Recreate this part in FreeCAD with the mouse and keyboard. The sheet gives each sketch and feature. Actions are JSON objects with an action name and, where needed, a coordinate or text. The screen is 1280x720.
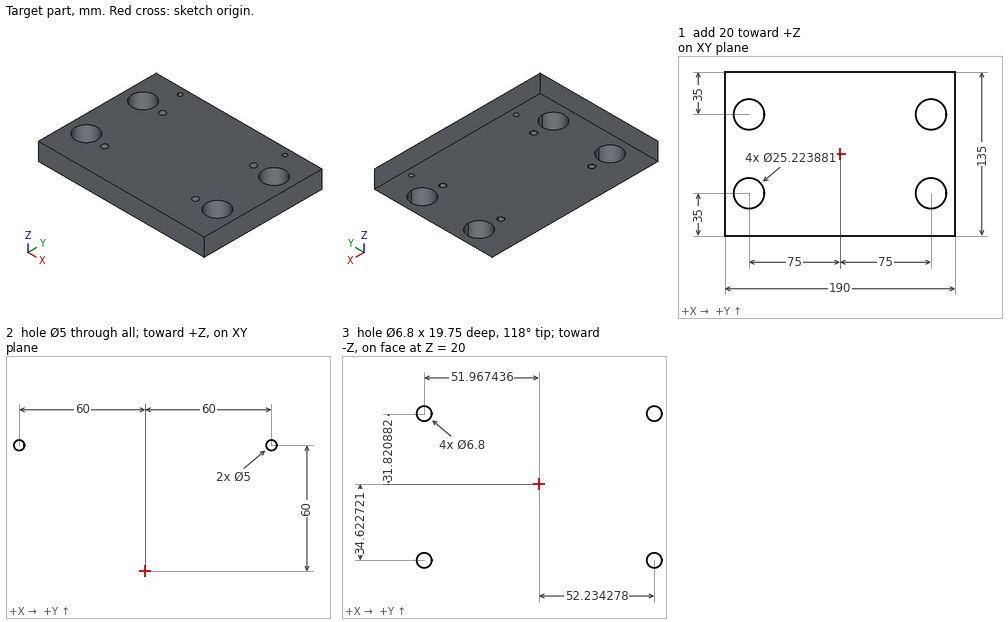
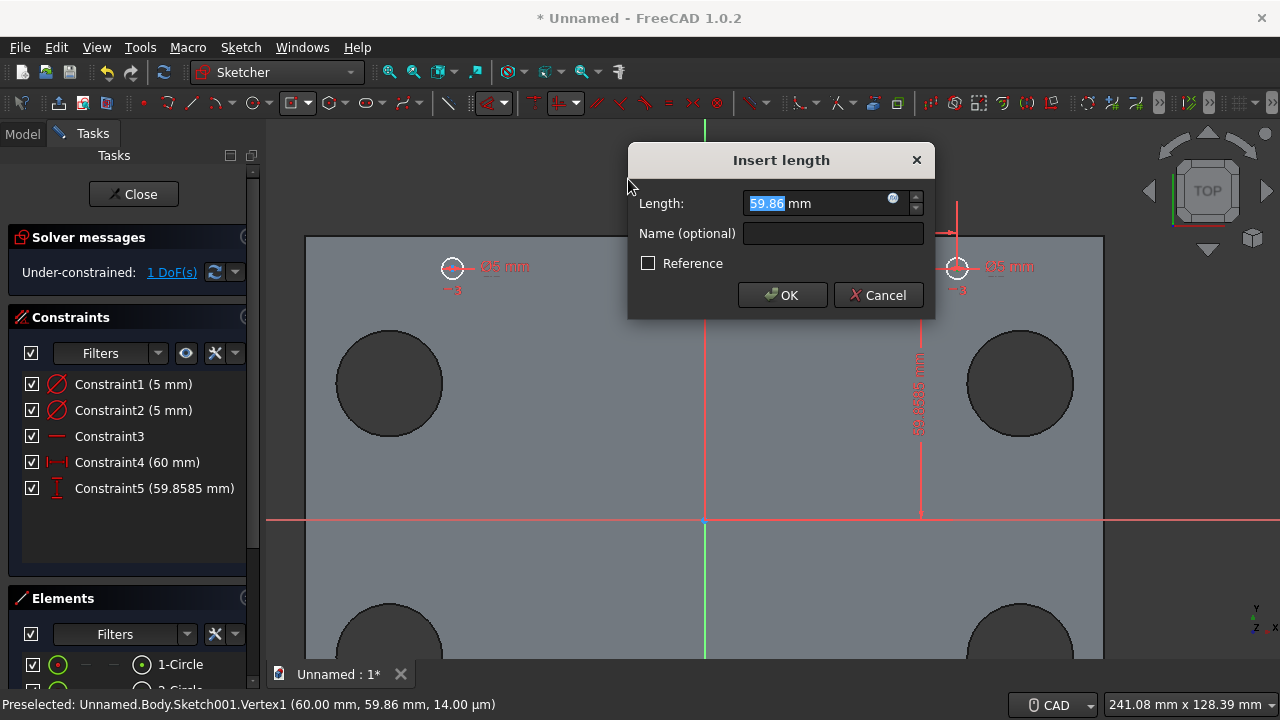
{"action": "type", "text": "60"}
{"action": "key", "text": "Return"}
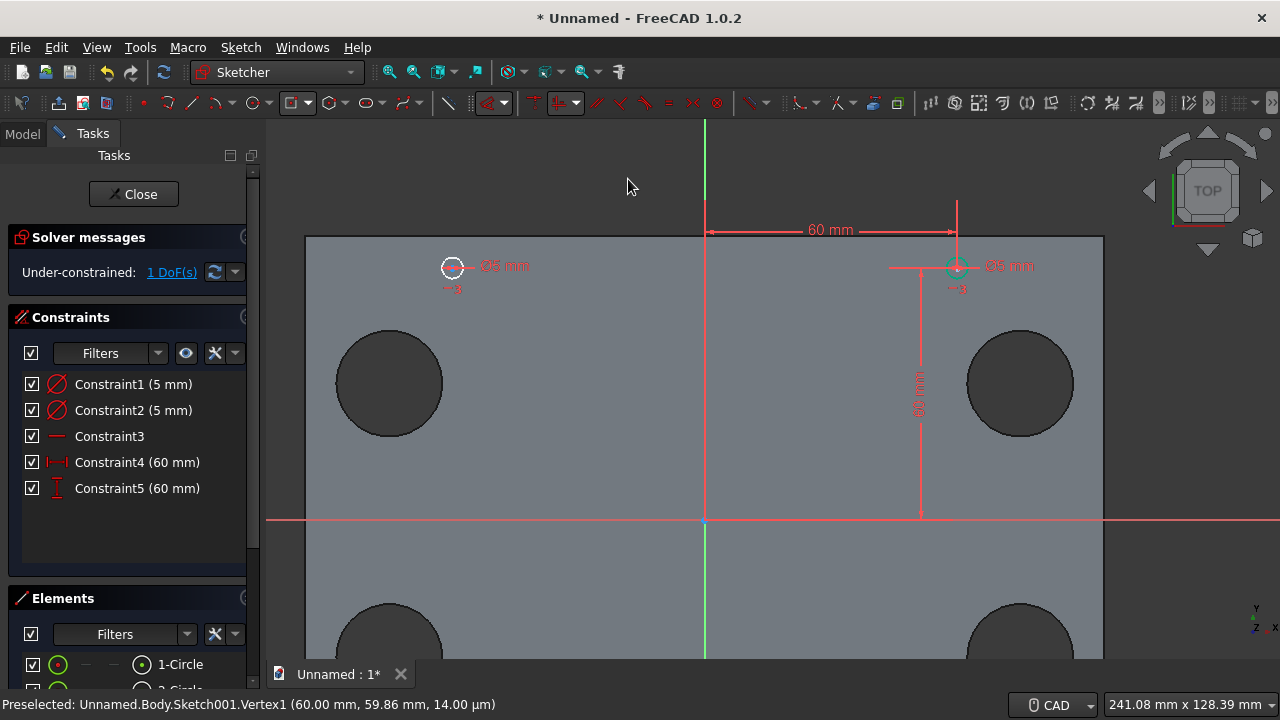
{"action": "left_click", "coordinate": [453, 268]}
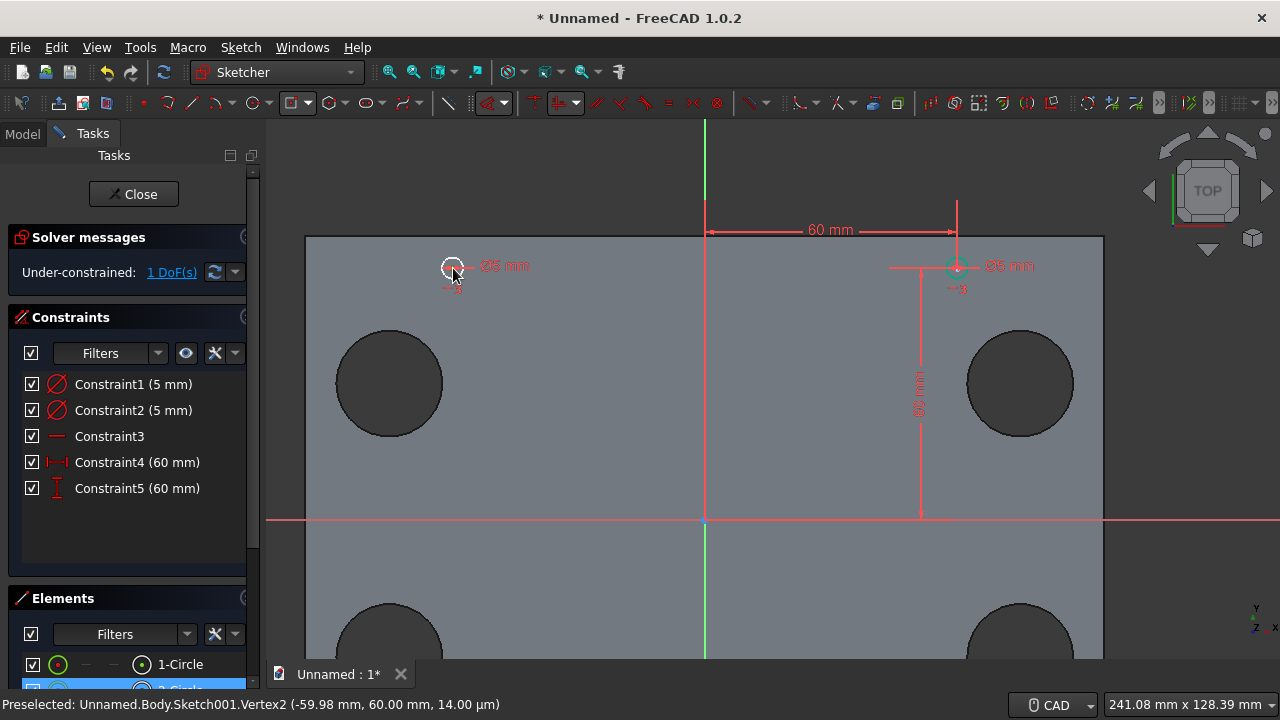
{"action": "left_click", "coordinate": [506, 104]}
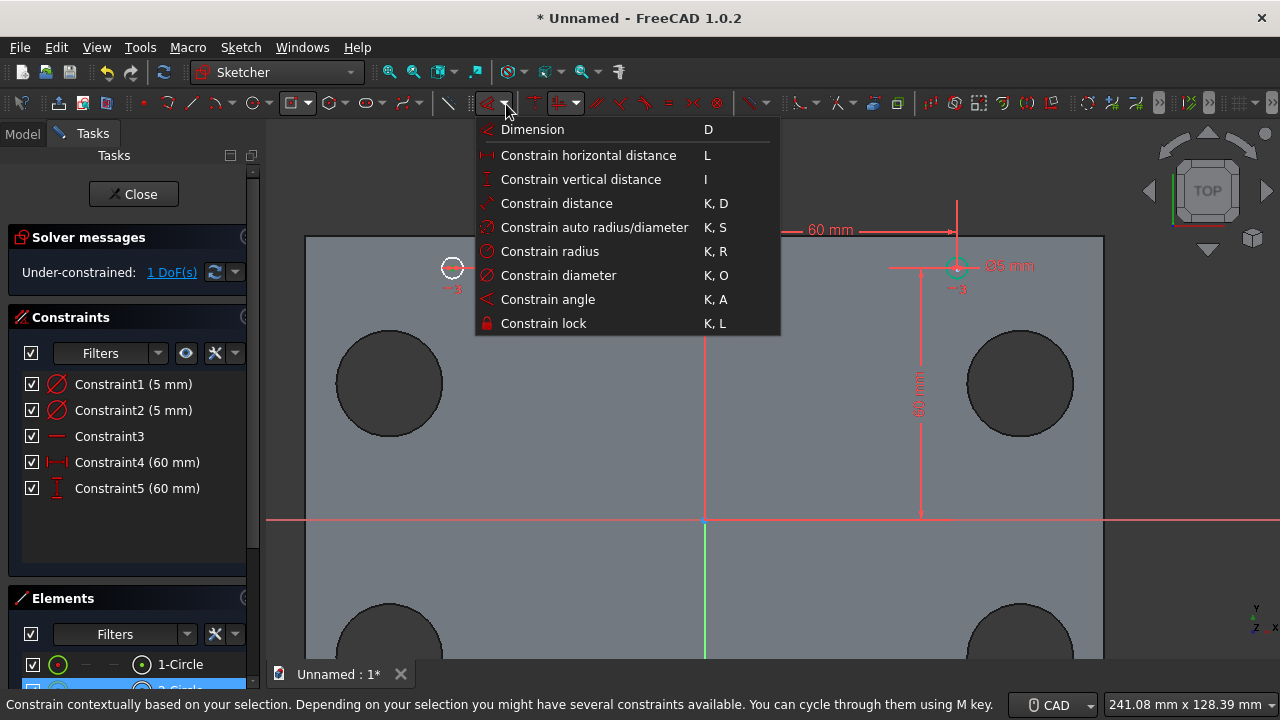
{"action": "left_click", "coordinate": [628, 155]}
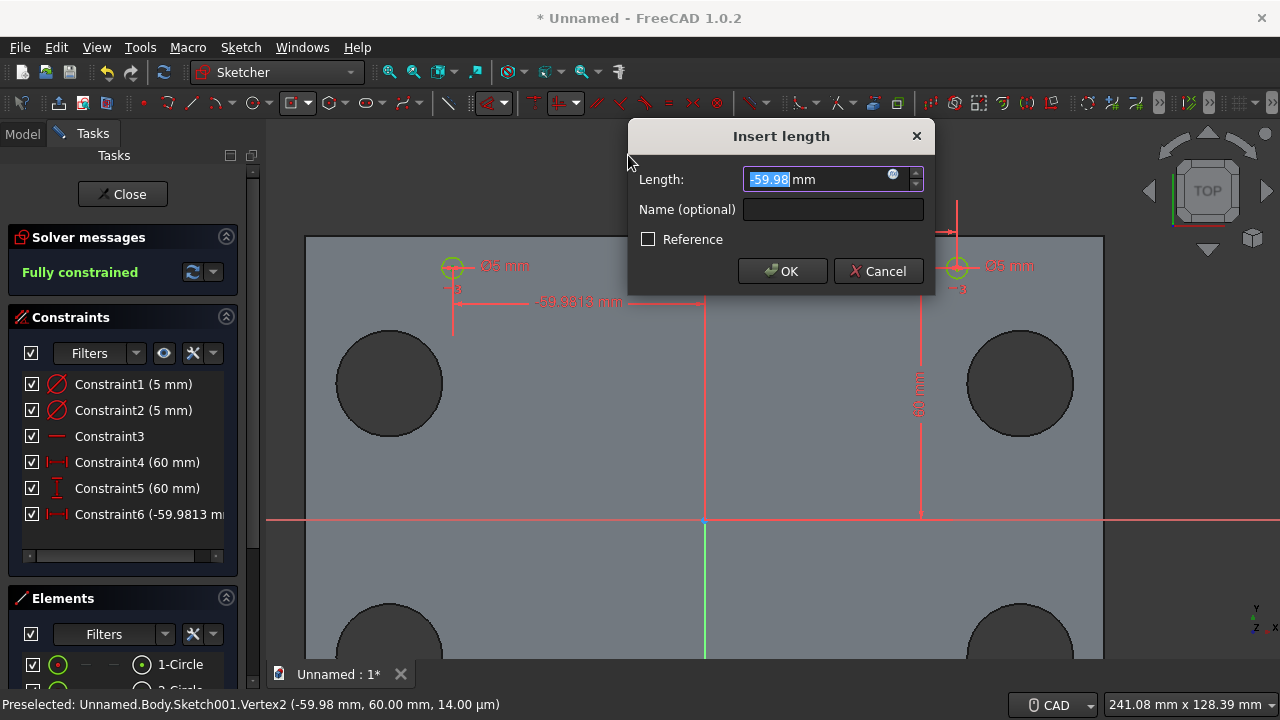
{"action": "type", "text": "-60"}
{"action": "key", "text": "Return"}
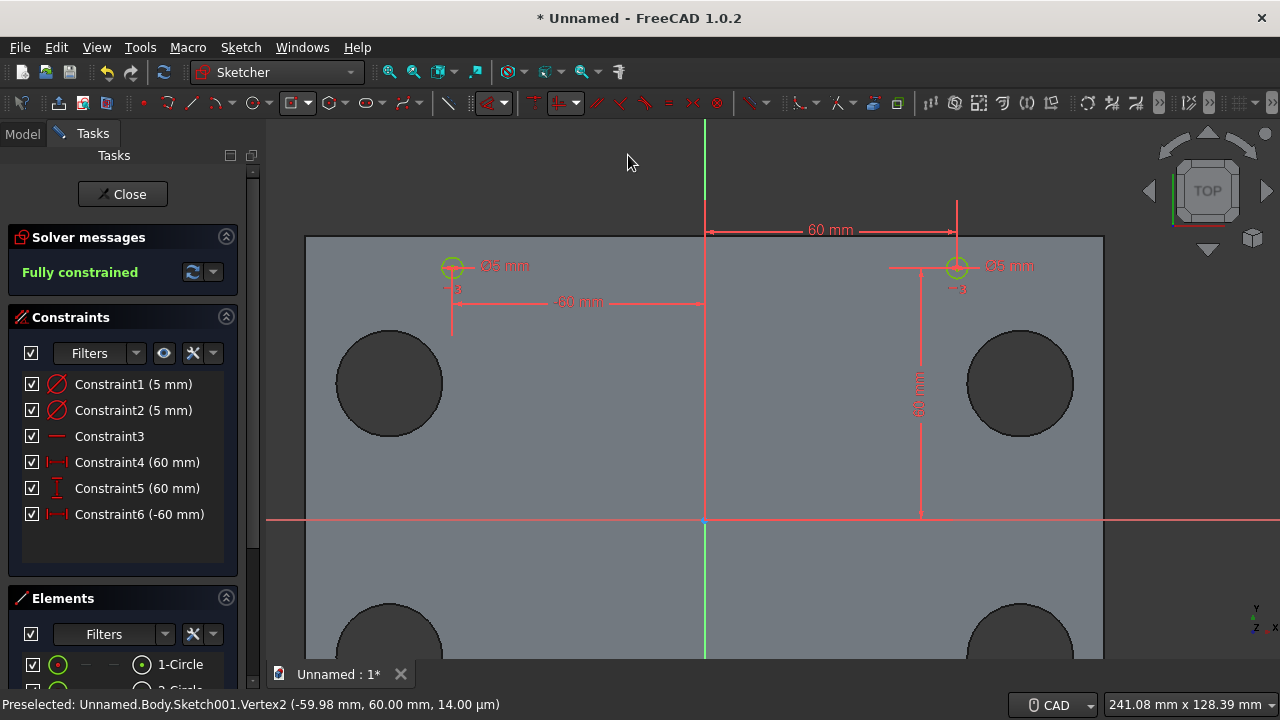
{"action": "left_click", "coordinate": [123, 194]}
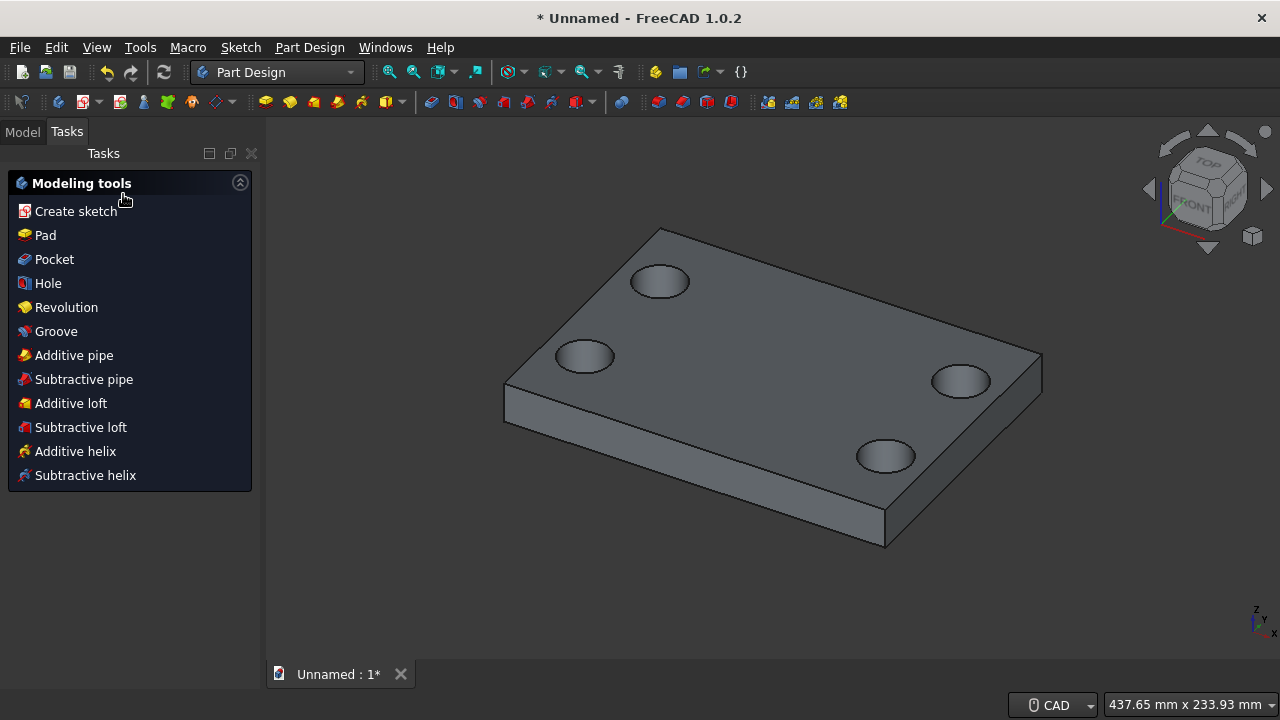
{"action": "left_click", "coordinate": [456, 102]}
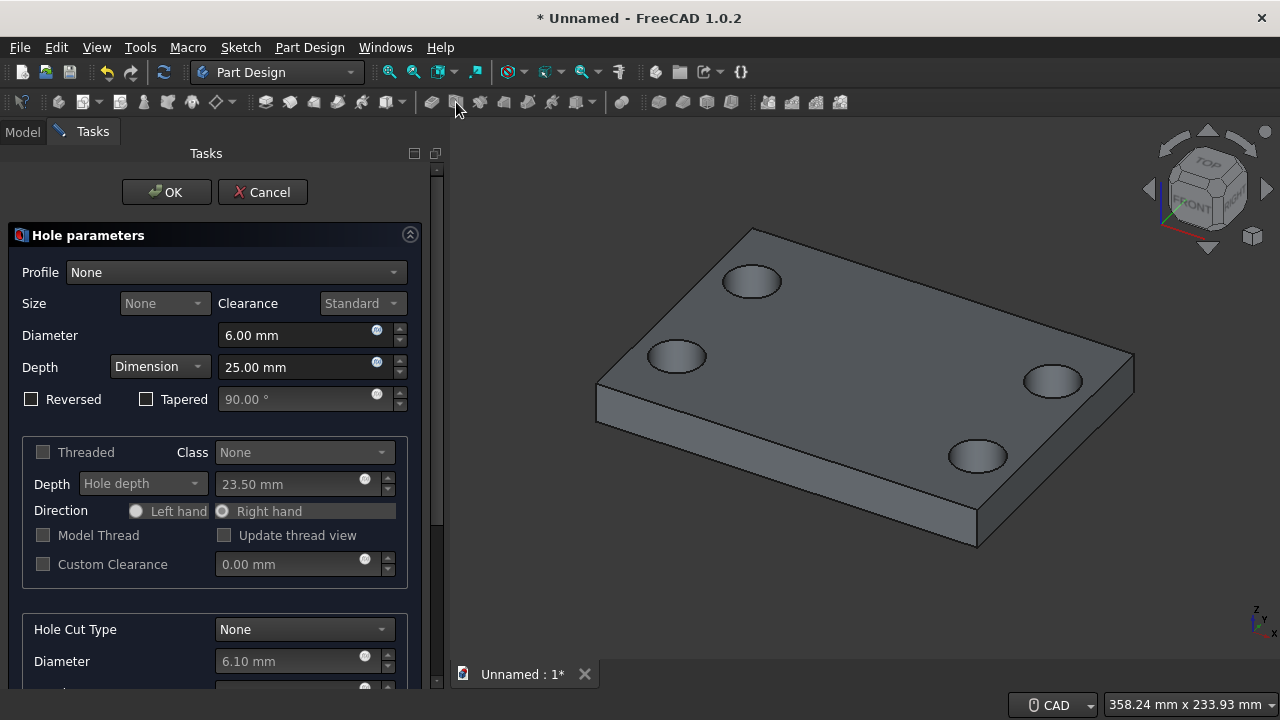
{"action": "triple_click", "coordinate": [305, 335]}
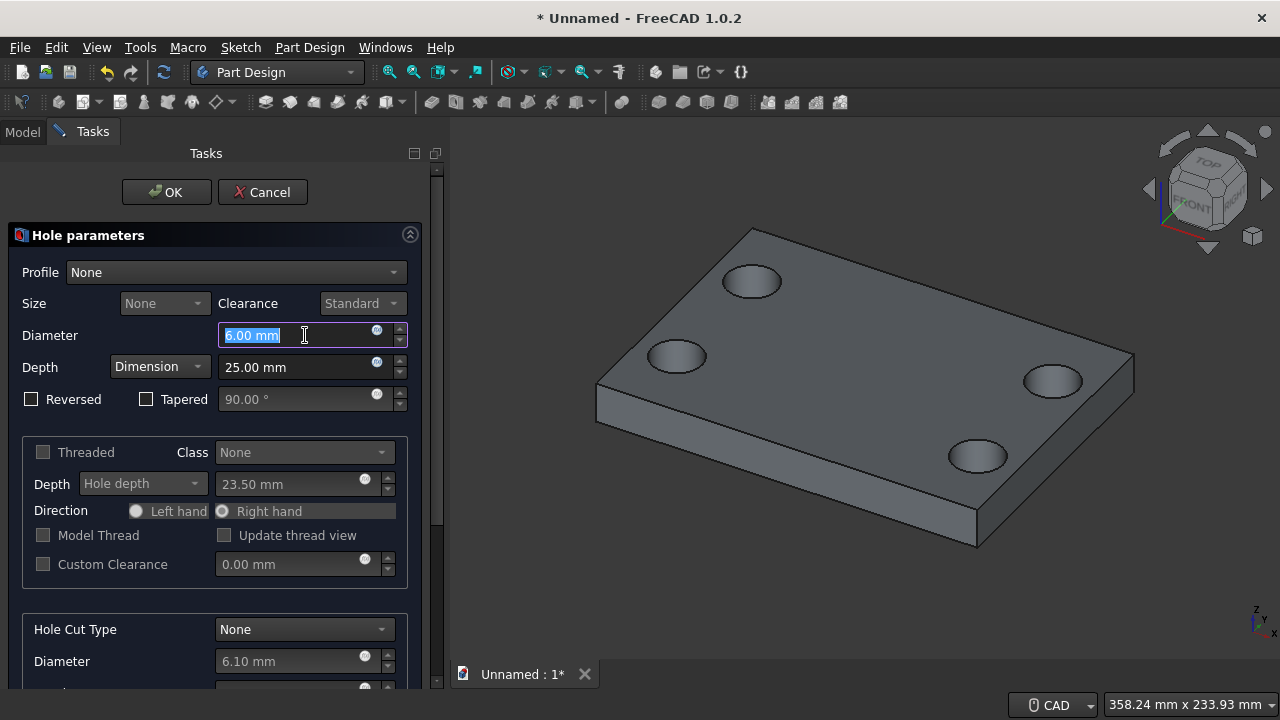
{"action": "type", "text": "5"}
{"action": "key", "text": "Tab"}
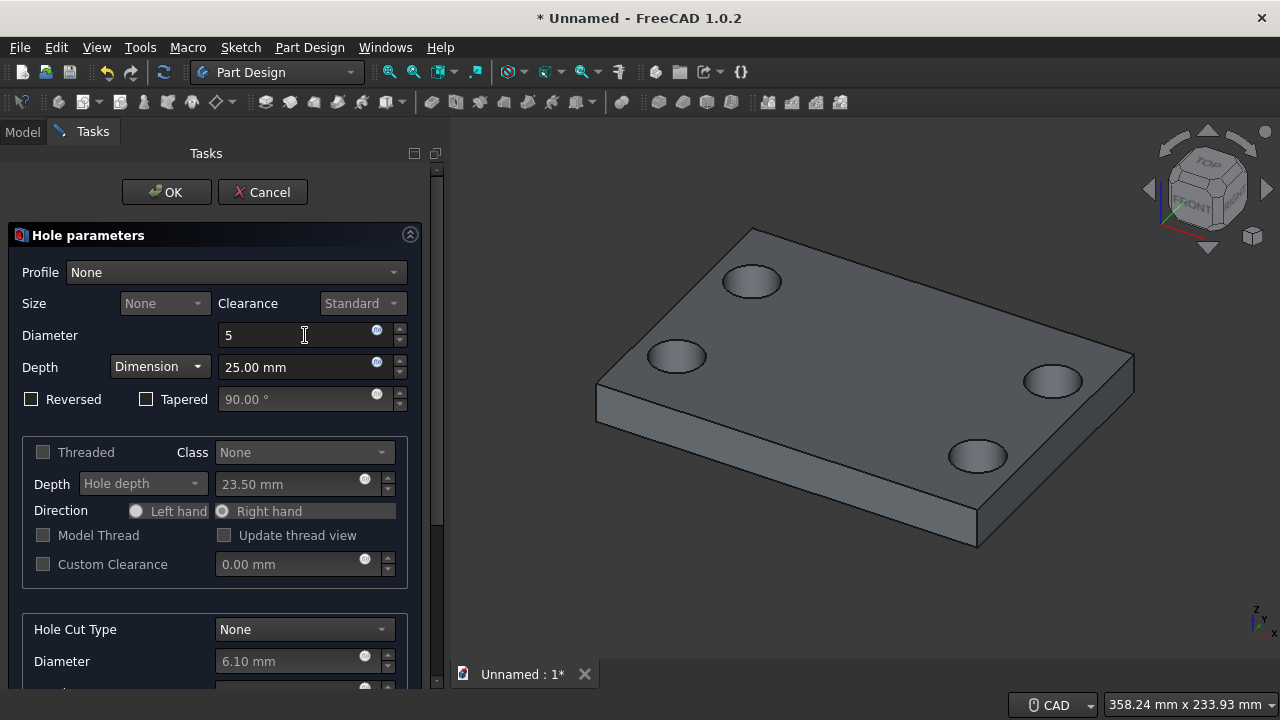
{"action": "left_click", "coordinate": [161, 366]}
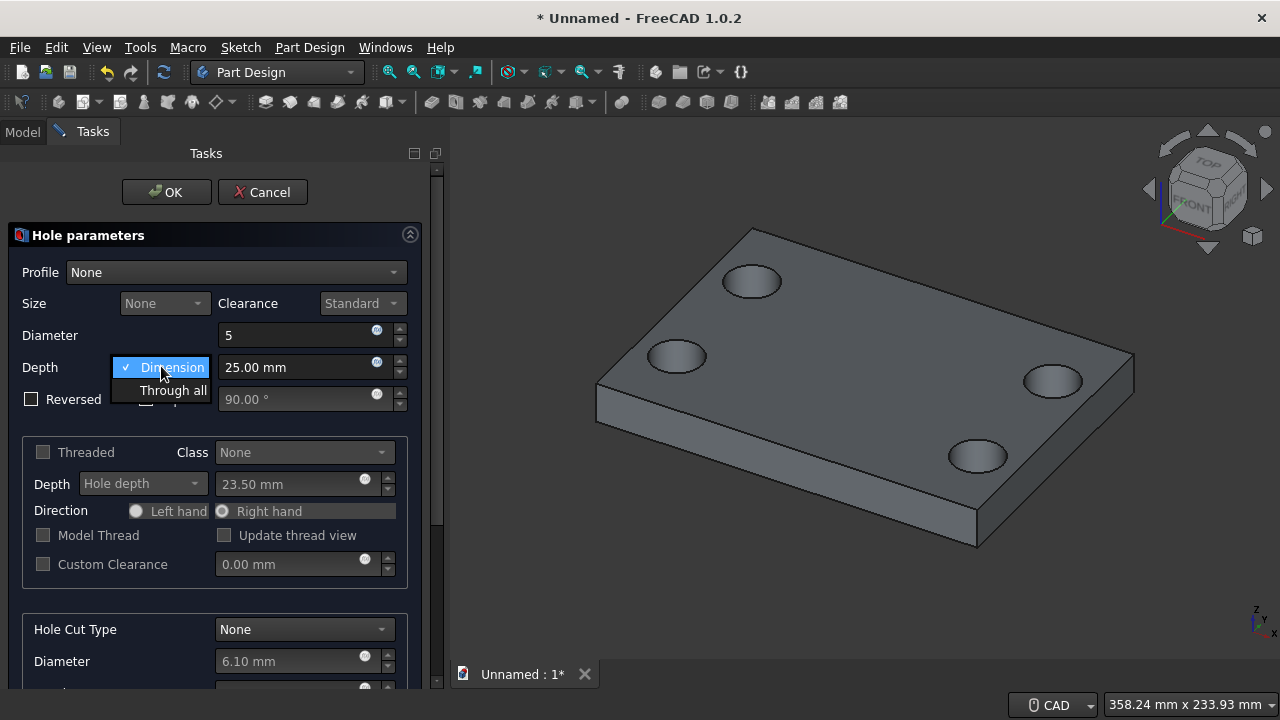
{"action": "left_click", "coordinate": [160, 390]}